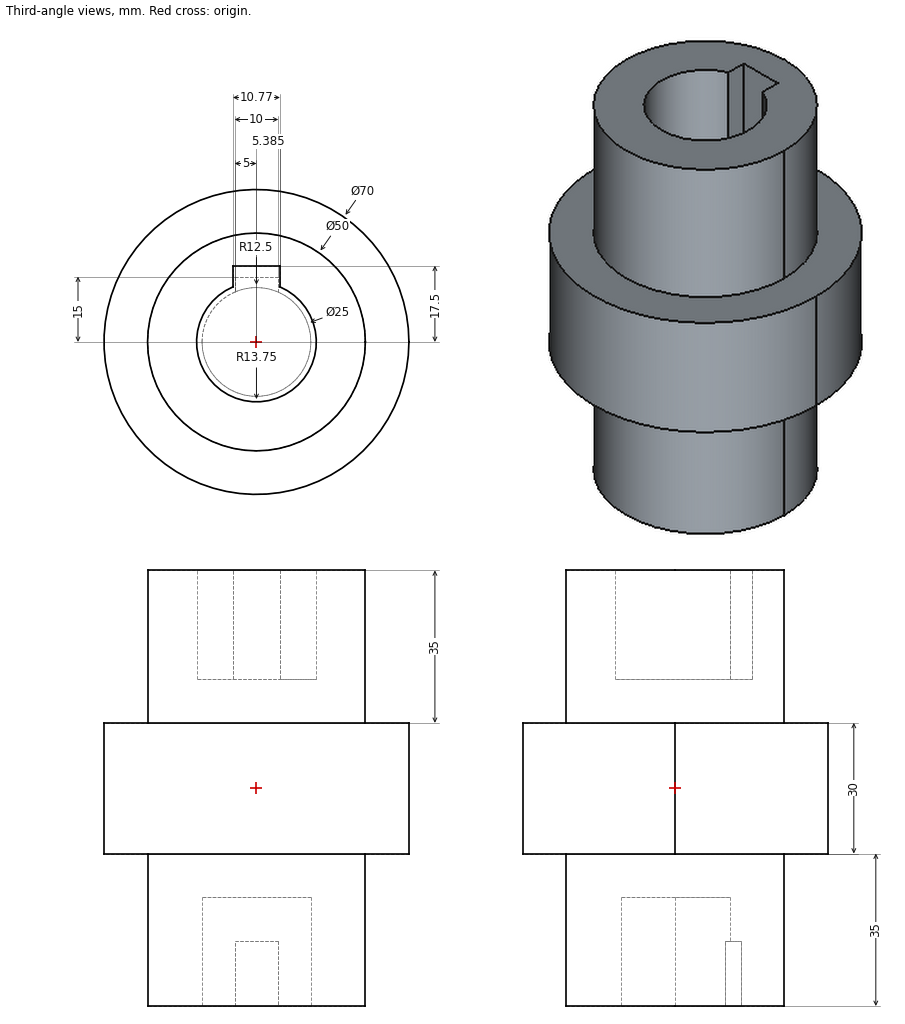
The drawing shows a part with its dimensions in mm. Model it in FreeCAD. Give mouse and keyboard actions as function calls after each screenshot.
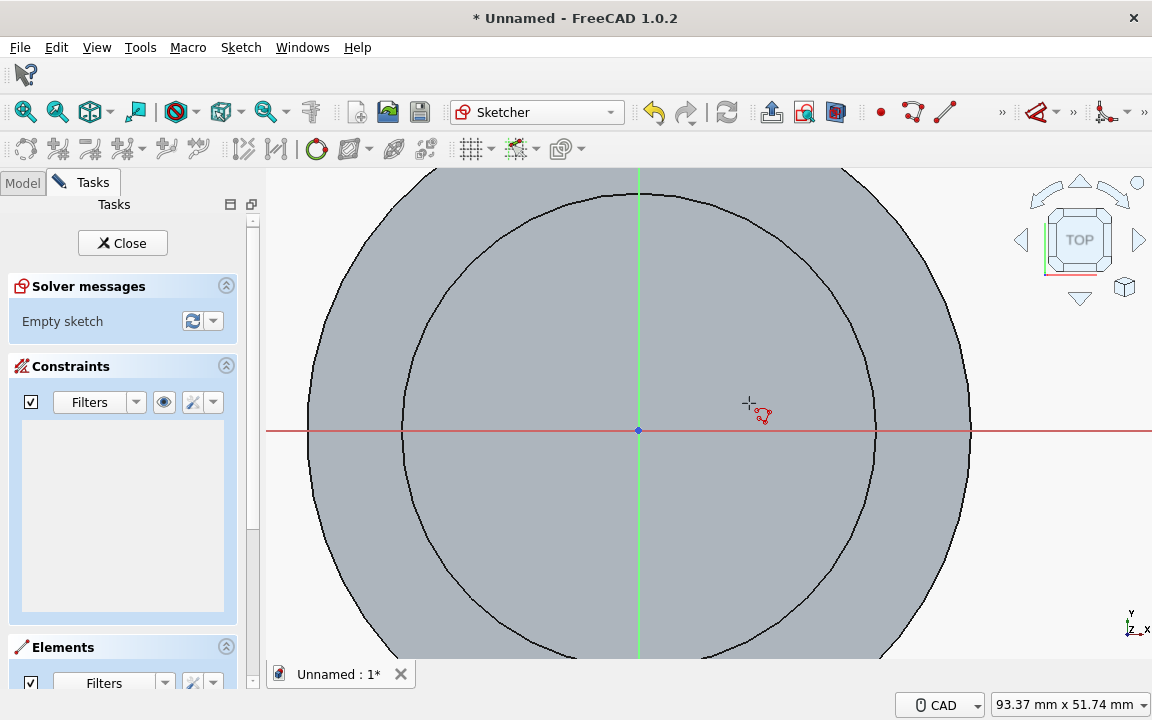
click(690, 311)
click(690, 265)
click(588, 265)
click(588, 311)
right_click(588, 311)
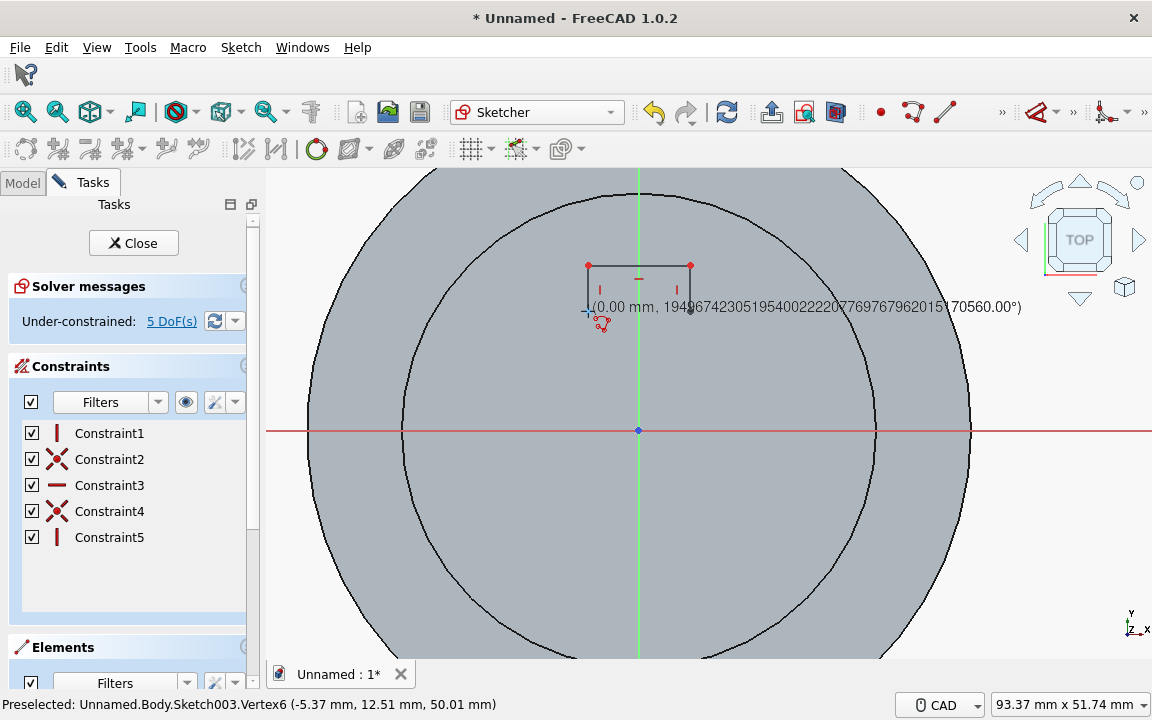
key(g)
key(3)
key(a)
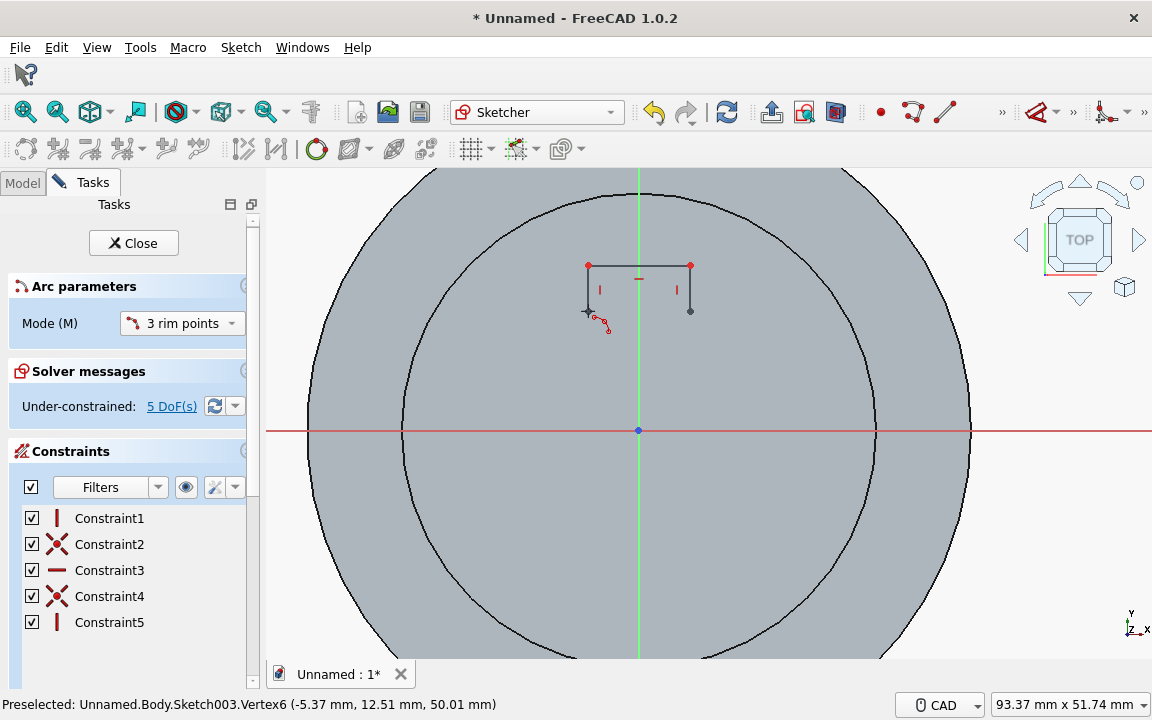
click(588, 312)
click(690, 312)
click(571, 542)
key(Escape)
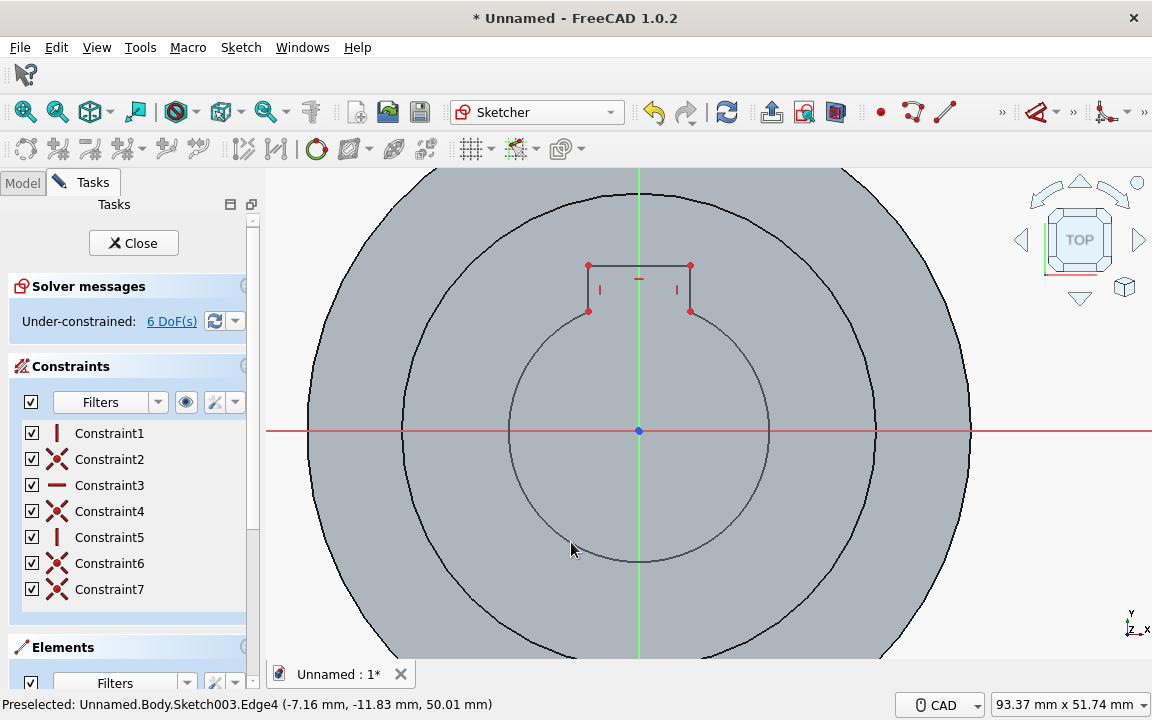
drag(629, 421, 649, 442)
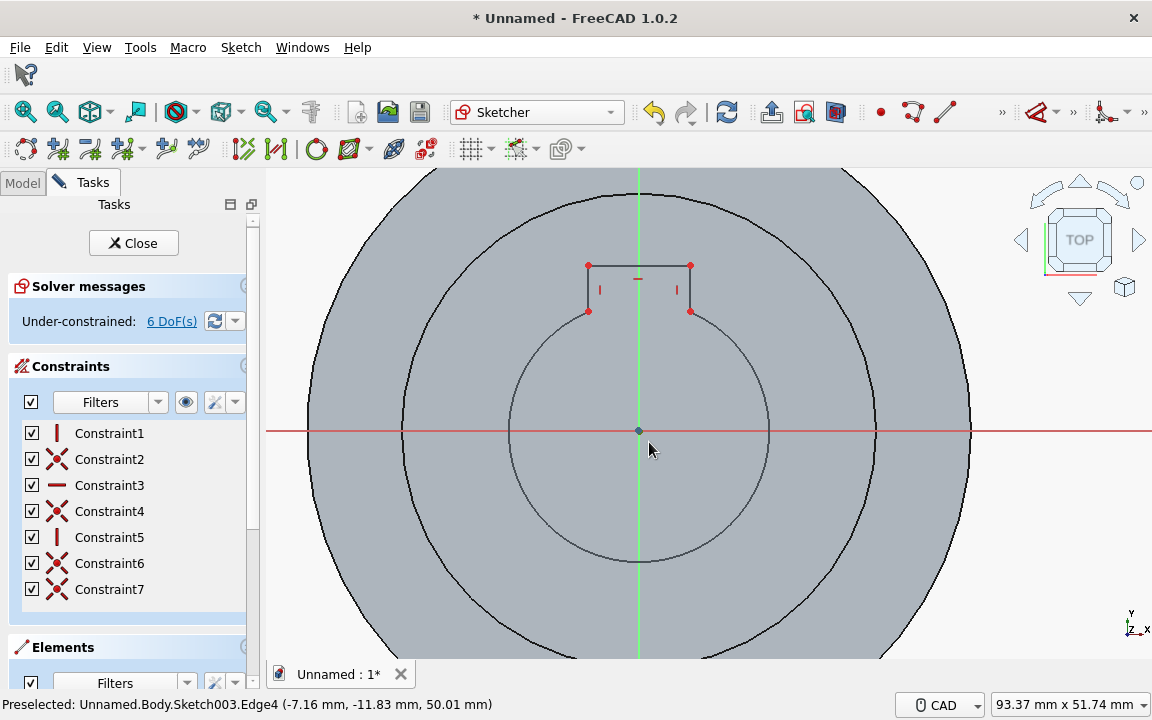
key(c)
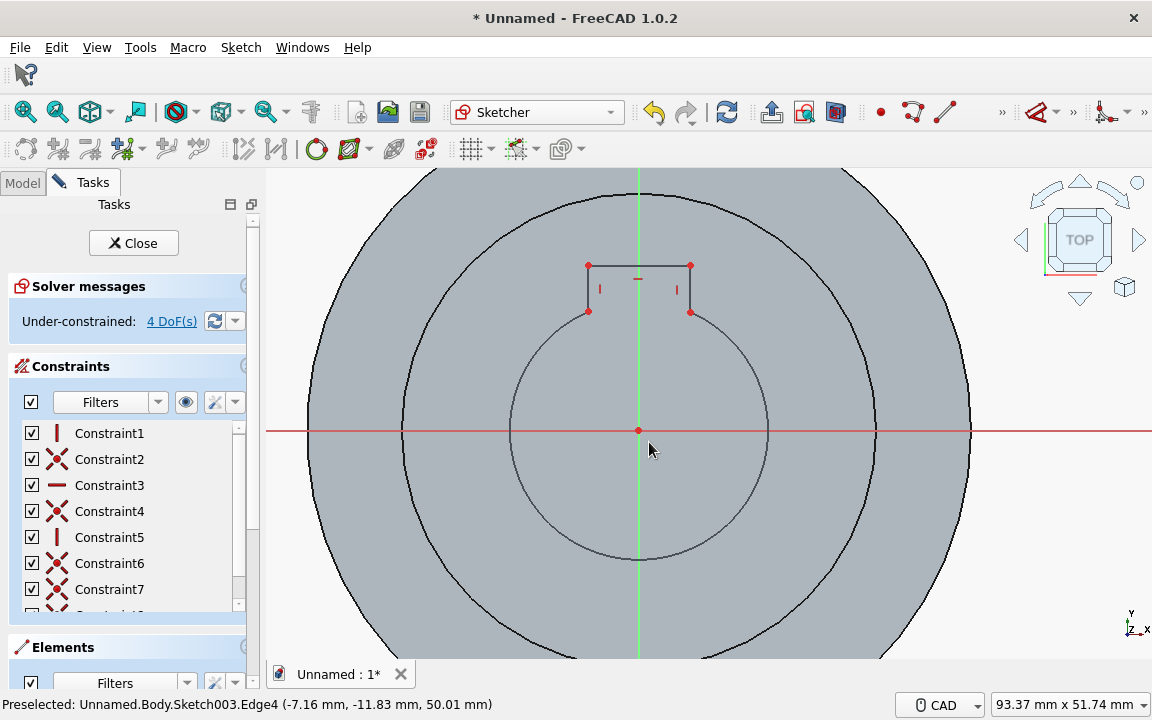
key(d)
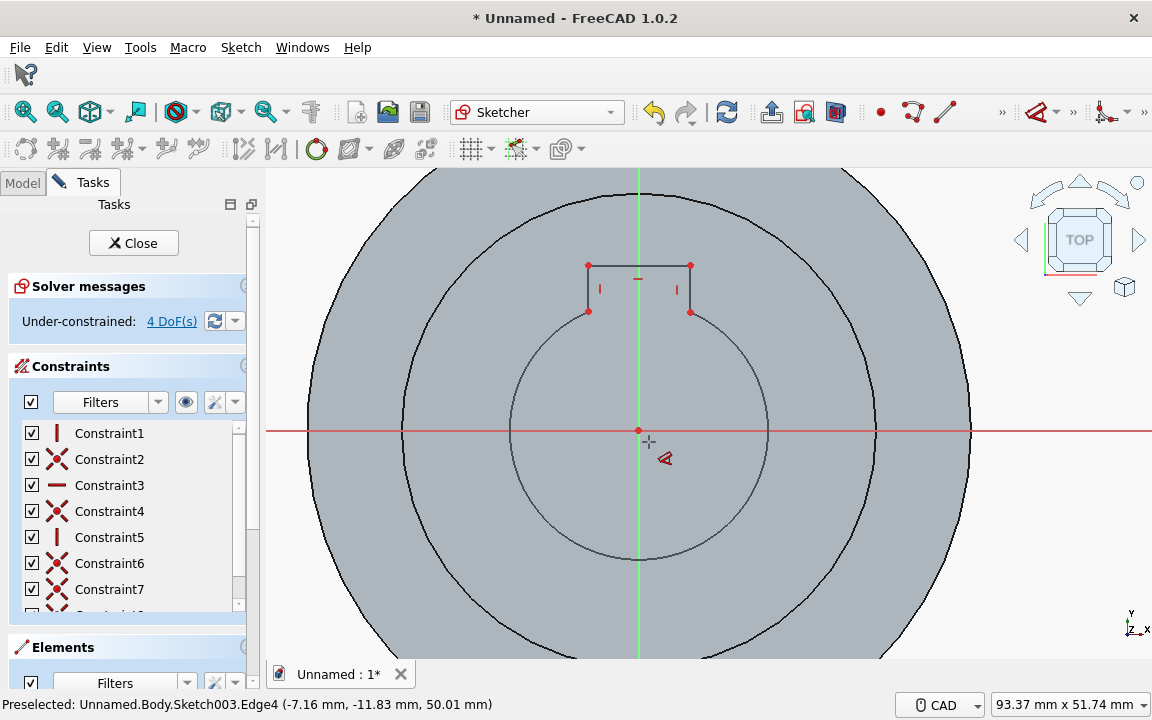
click(524, 490)
click(496, 505)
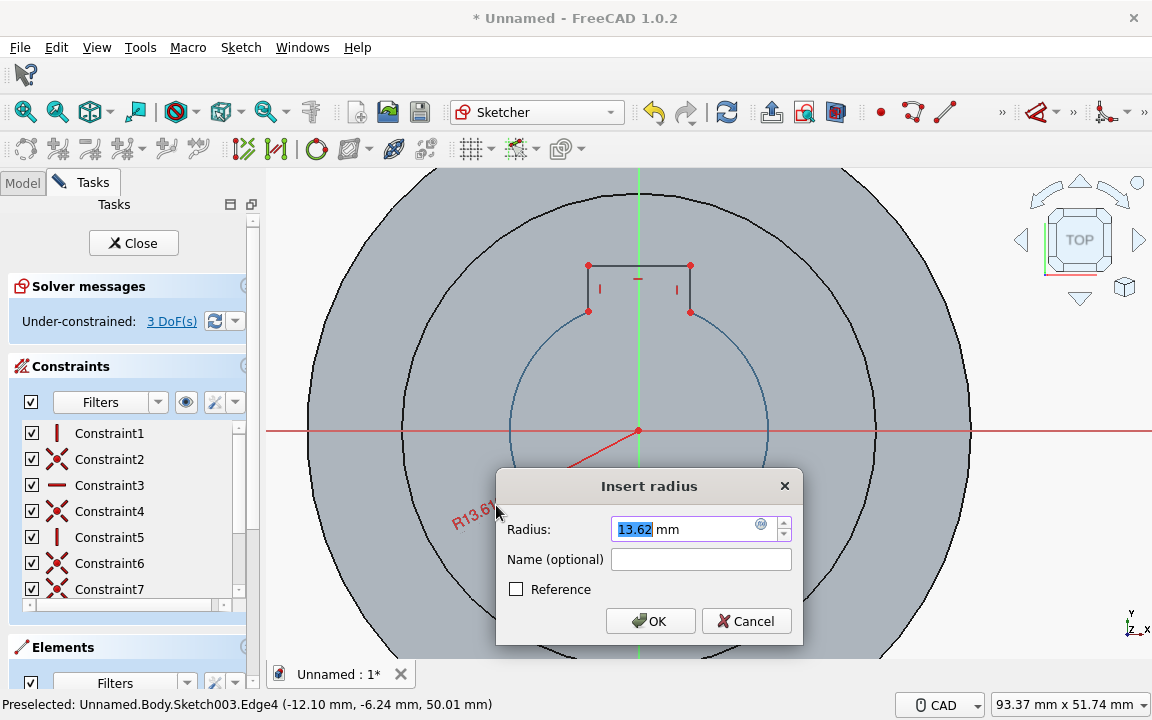
text(13.75)
key(Return)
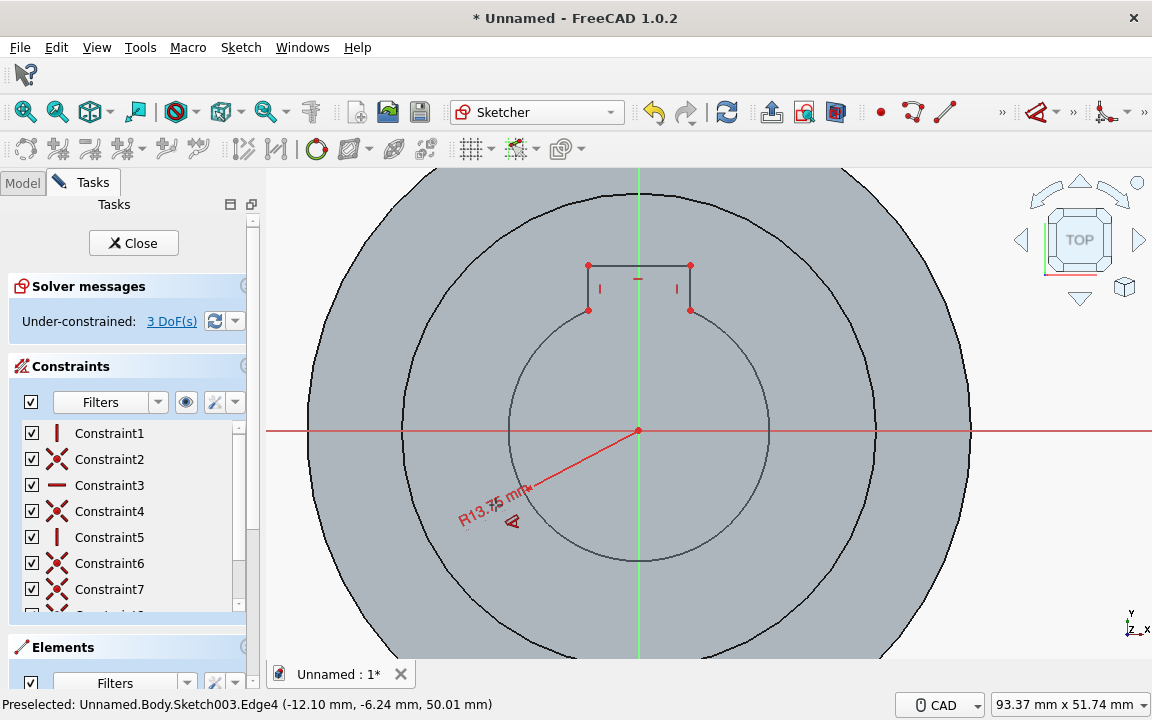
click(659, 266)
click(616, 232)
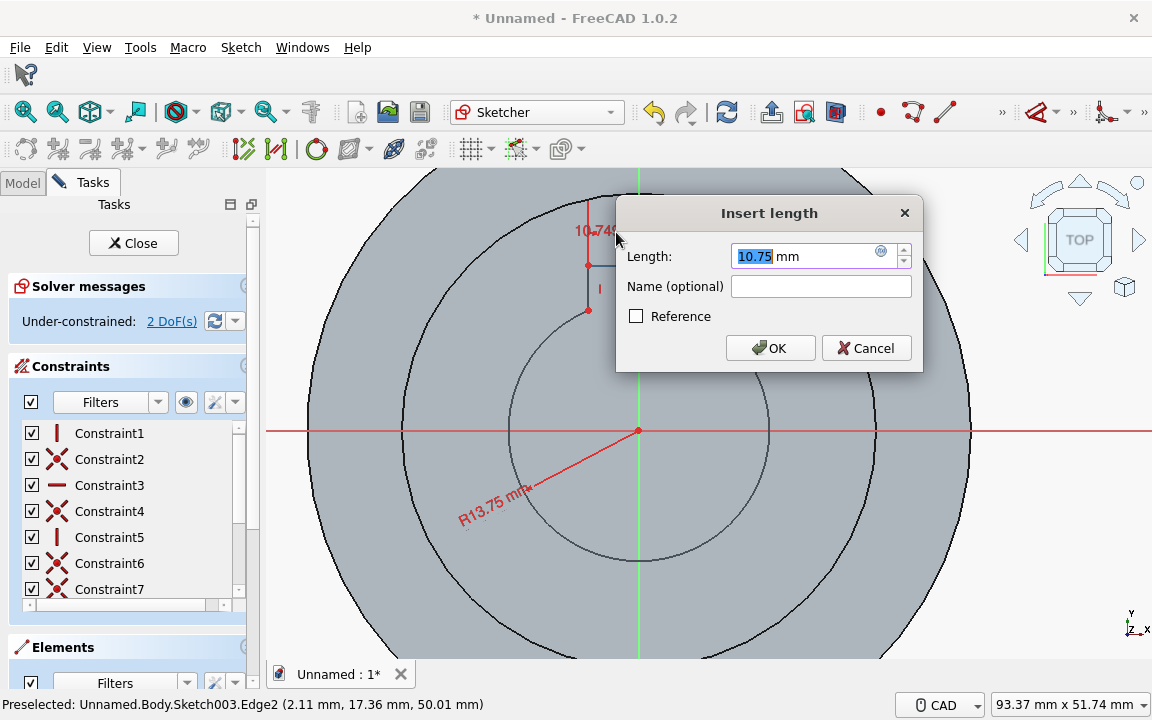
text(10.77)
key(Return)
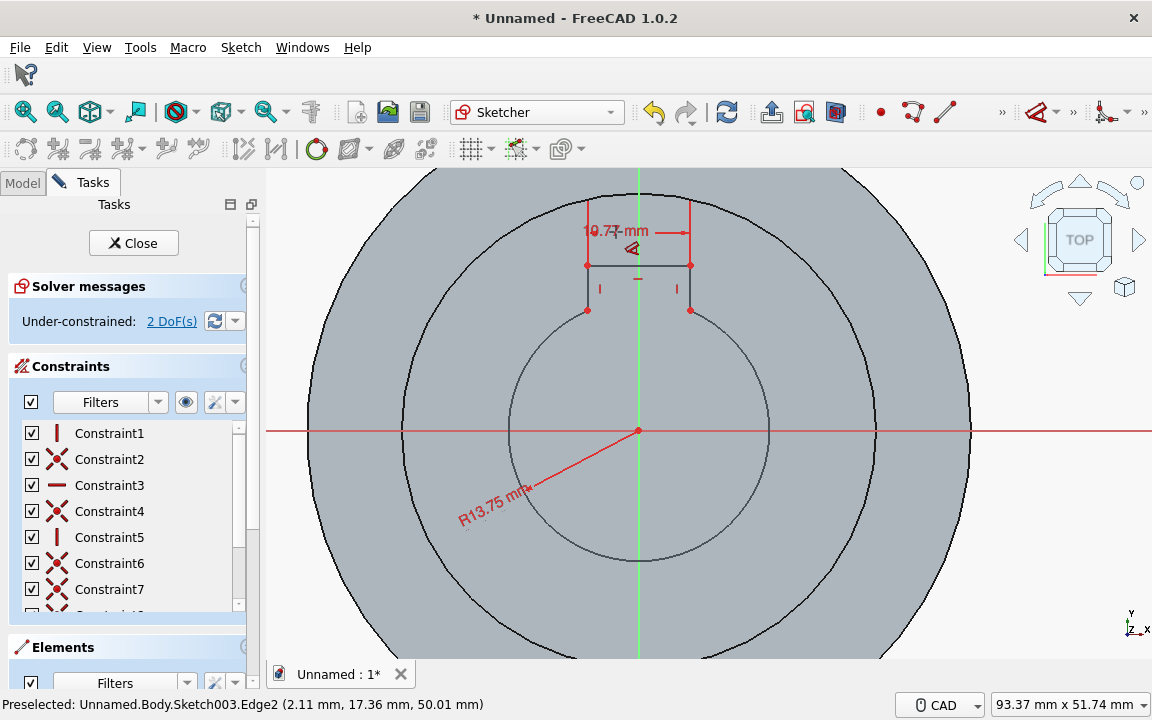
click(690, 266)
click(724, 310)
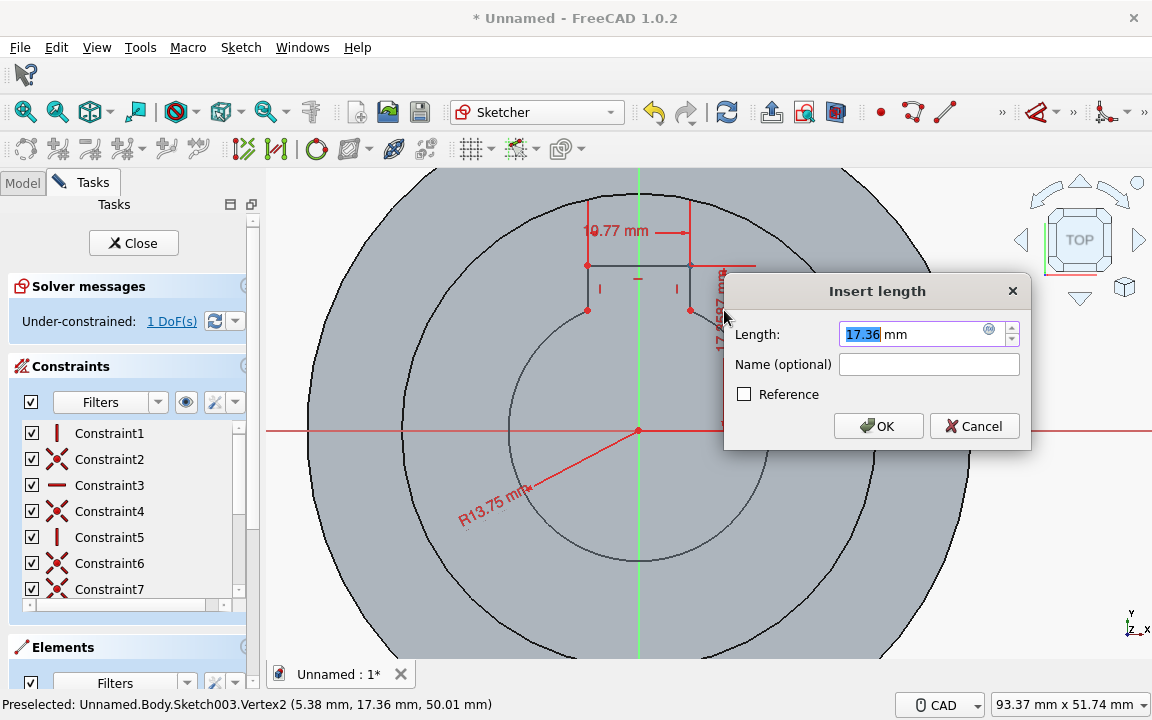
text(17.5)
key(Return)